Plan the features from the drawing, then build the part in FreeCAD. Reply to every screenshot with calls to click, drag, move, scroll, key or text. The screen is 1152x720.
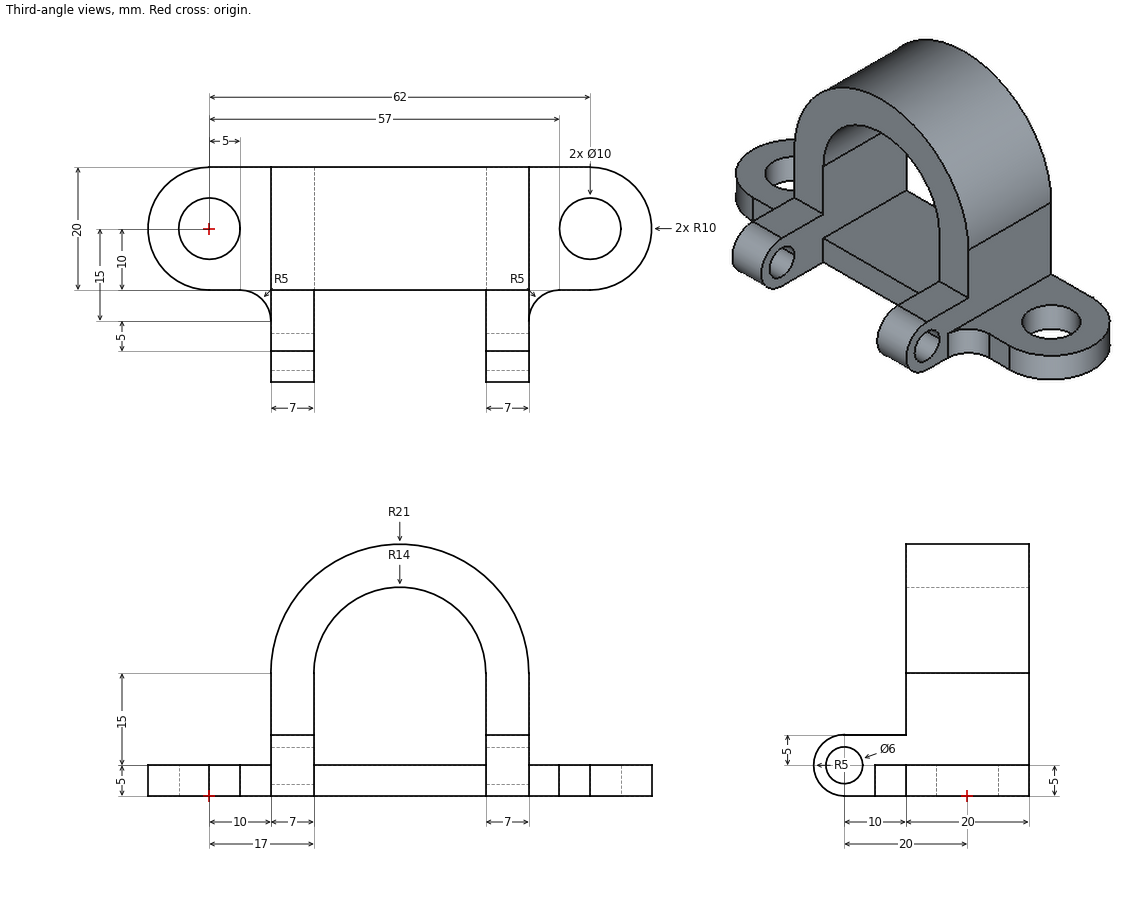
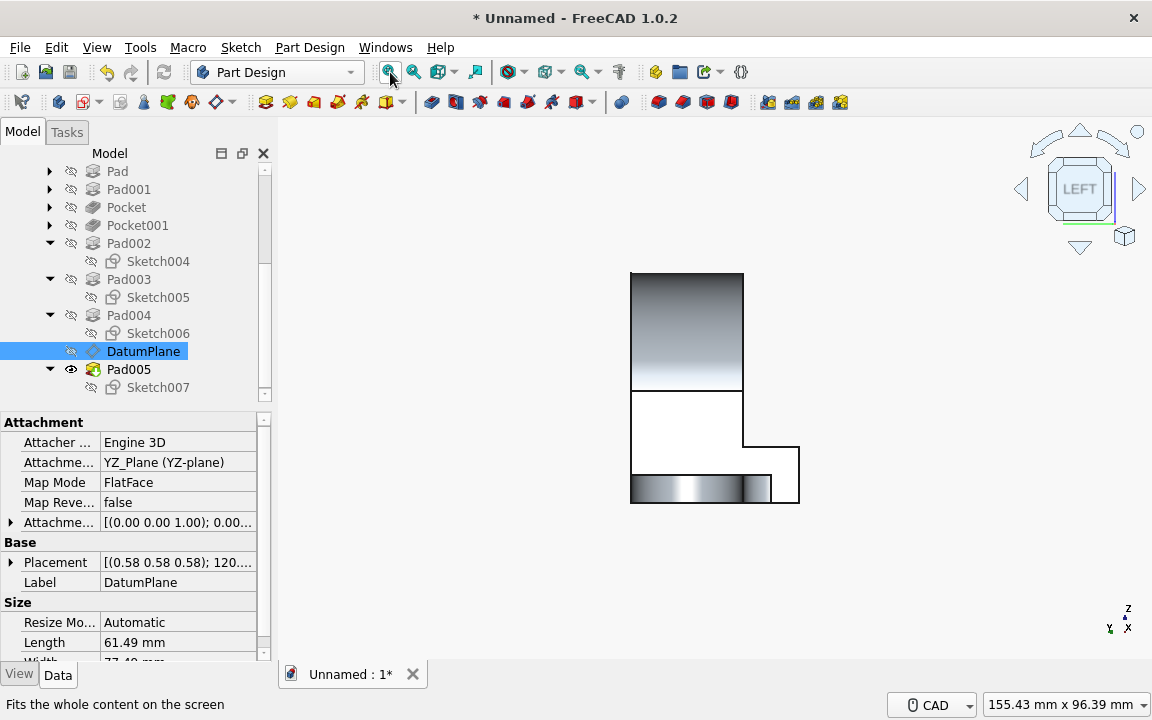
click(691, 430)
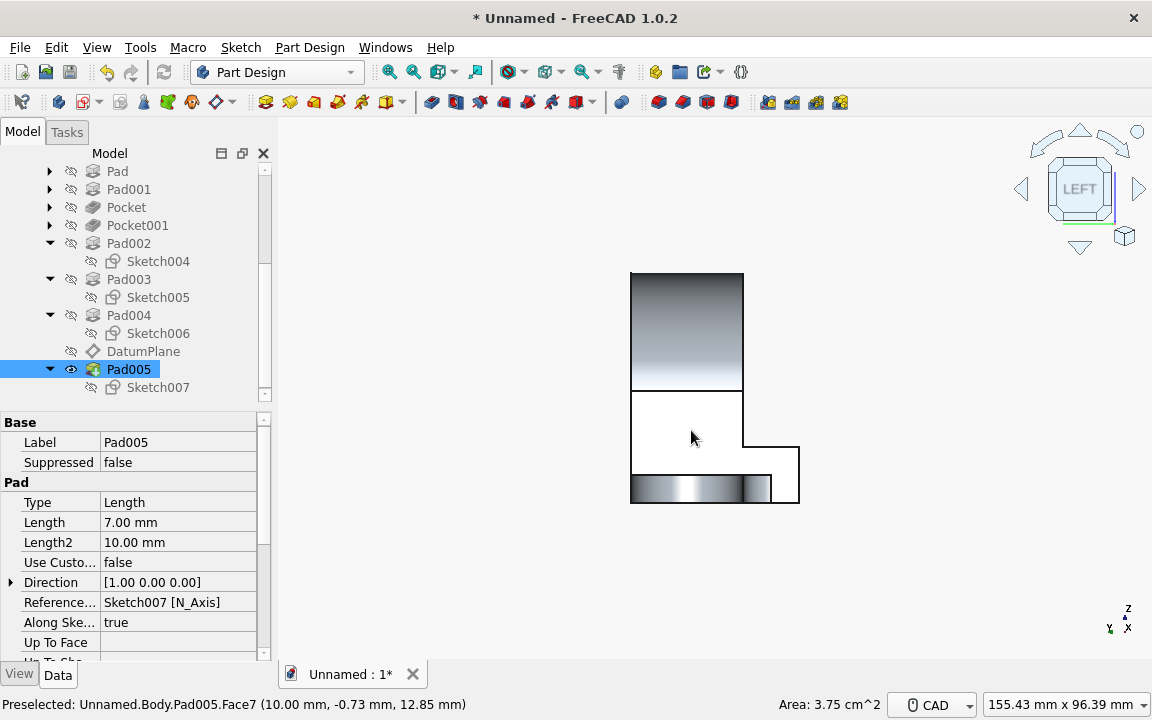
click(84, 102)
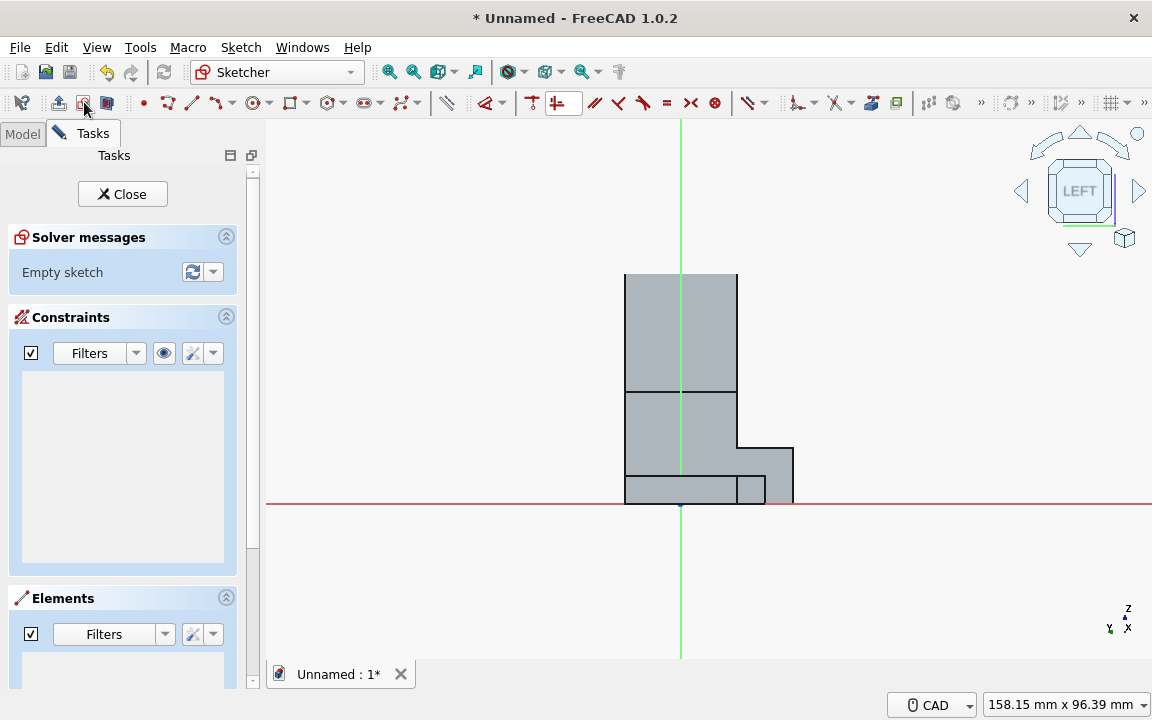
click(108, 104)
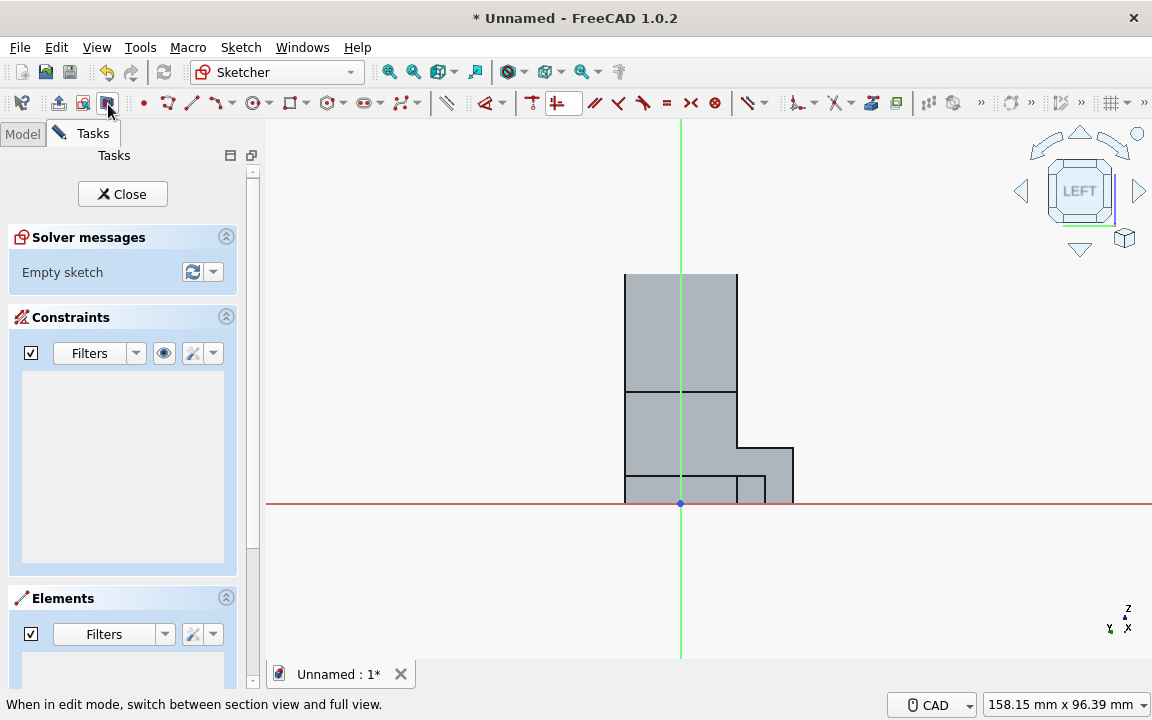
scroll(840, 493, up, 9)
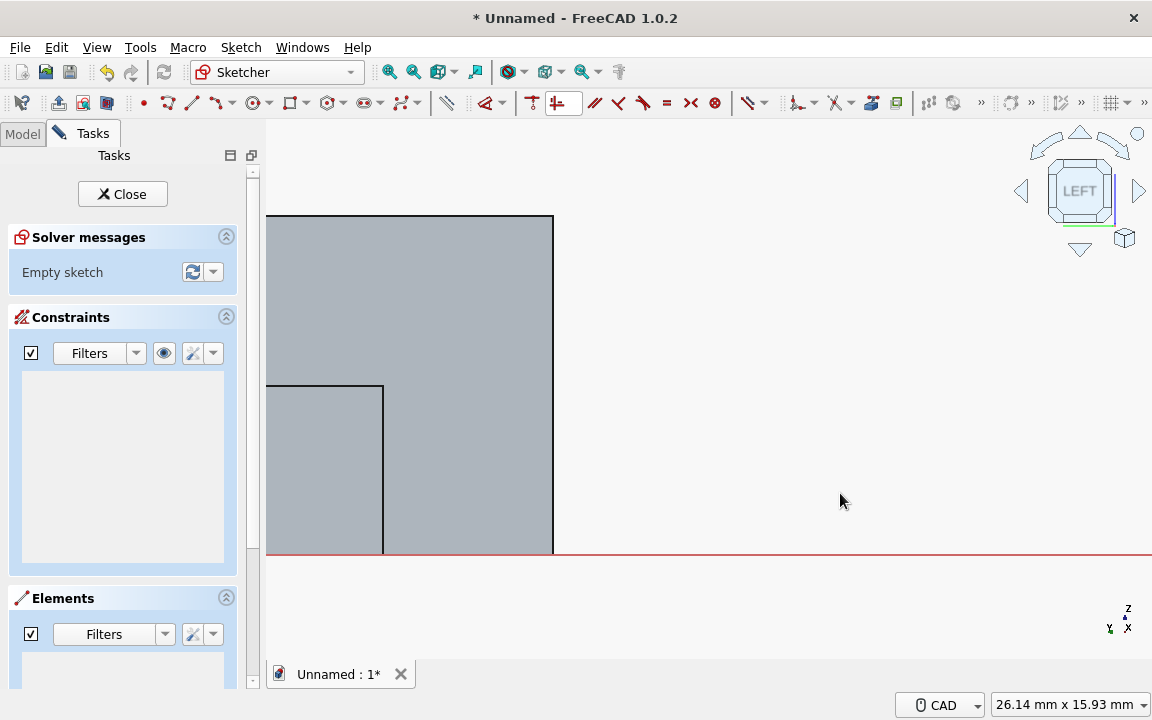
click(192, 104)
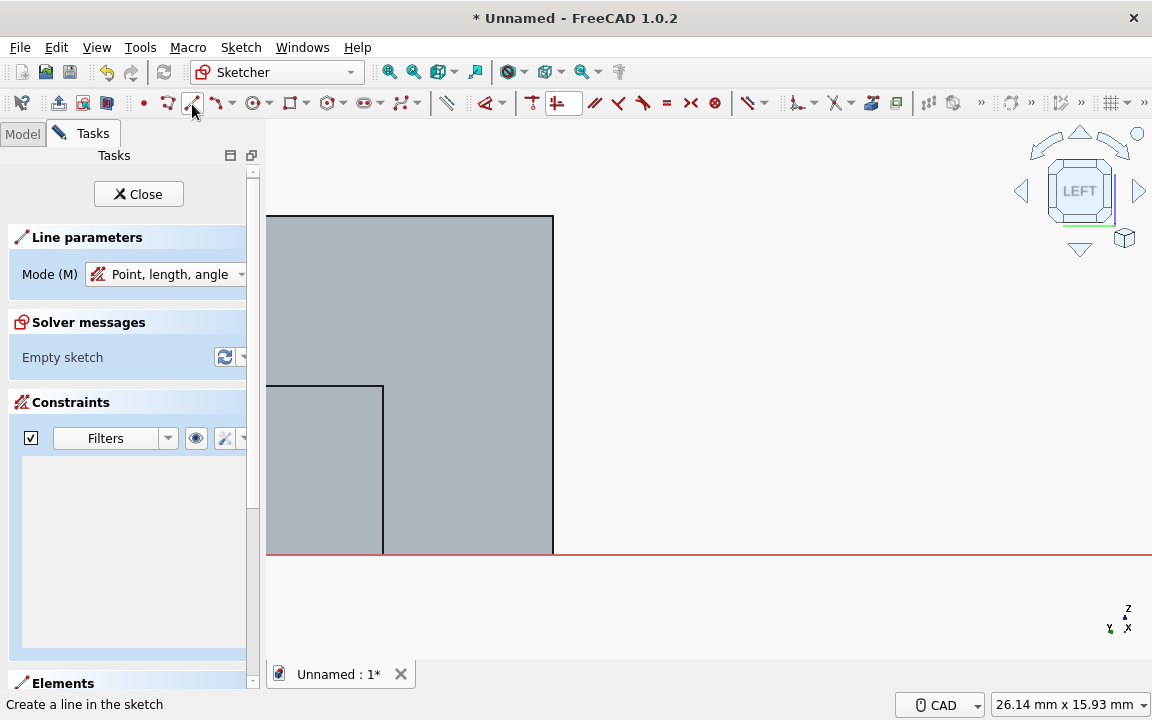
click(553, 216)
click(553, 555)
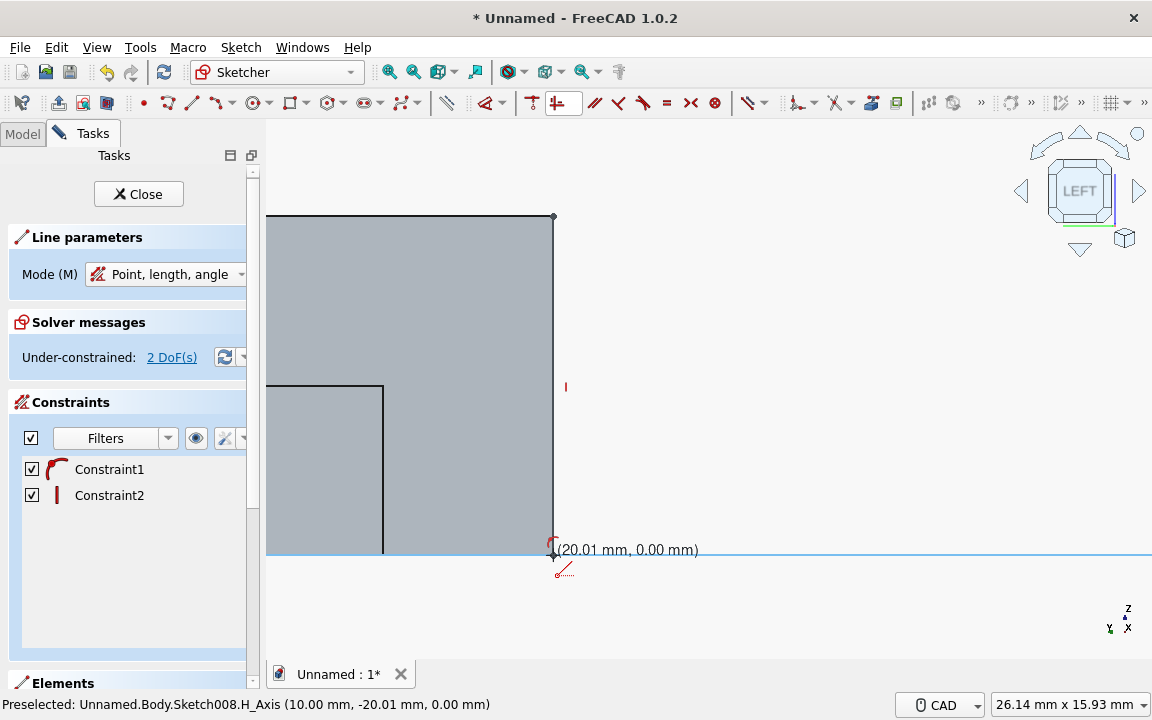
click(216, 104)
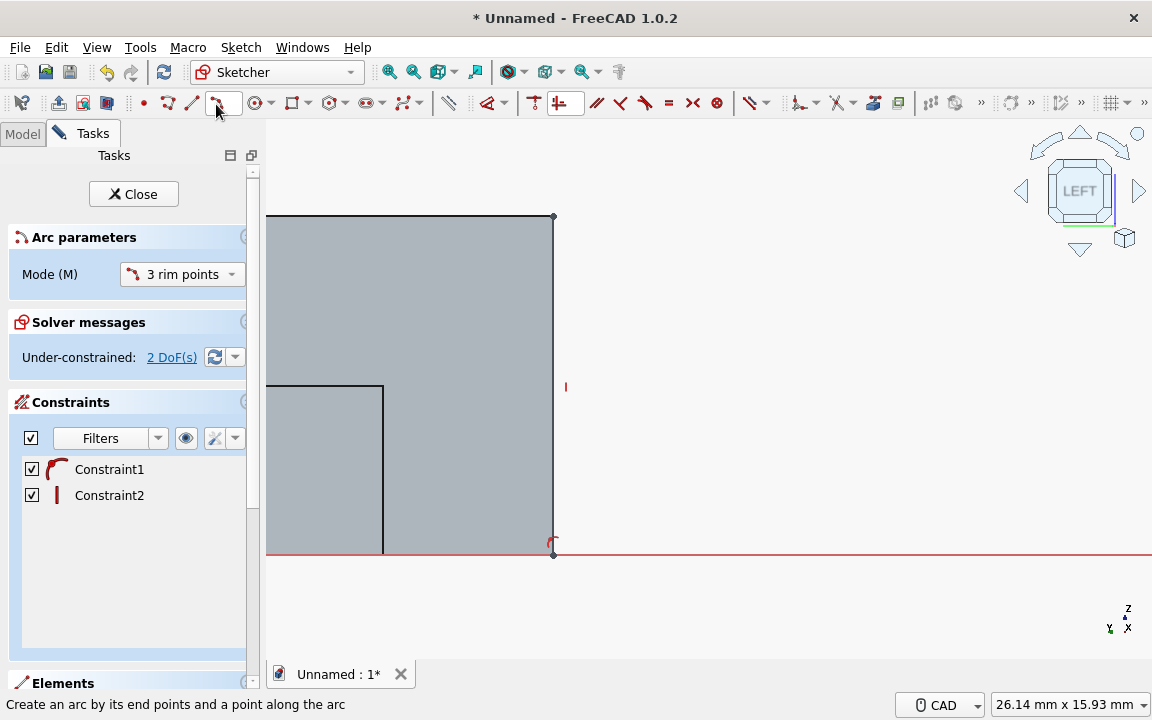
click(553, 555)
click(553, 217)
click(722, 386)
key(Escape)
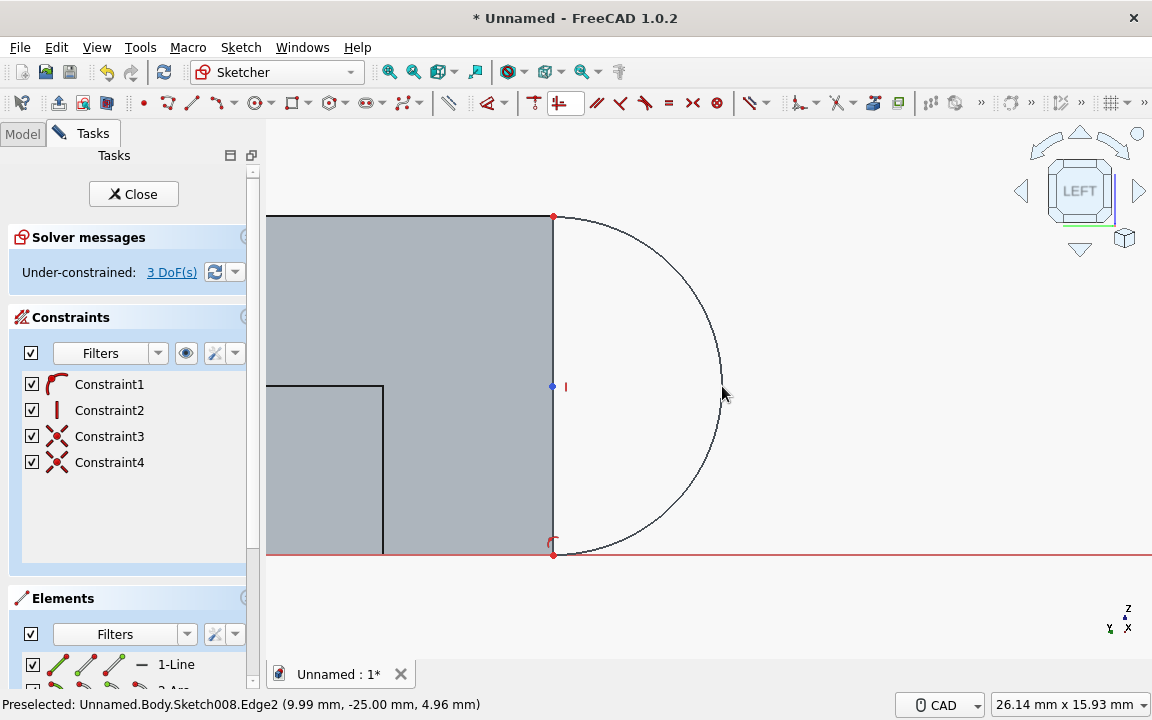
click(488, 104)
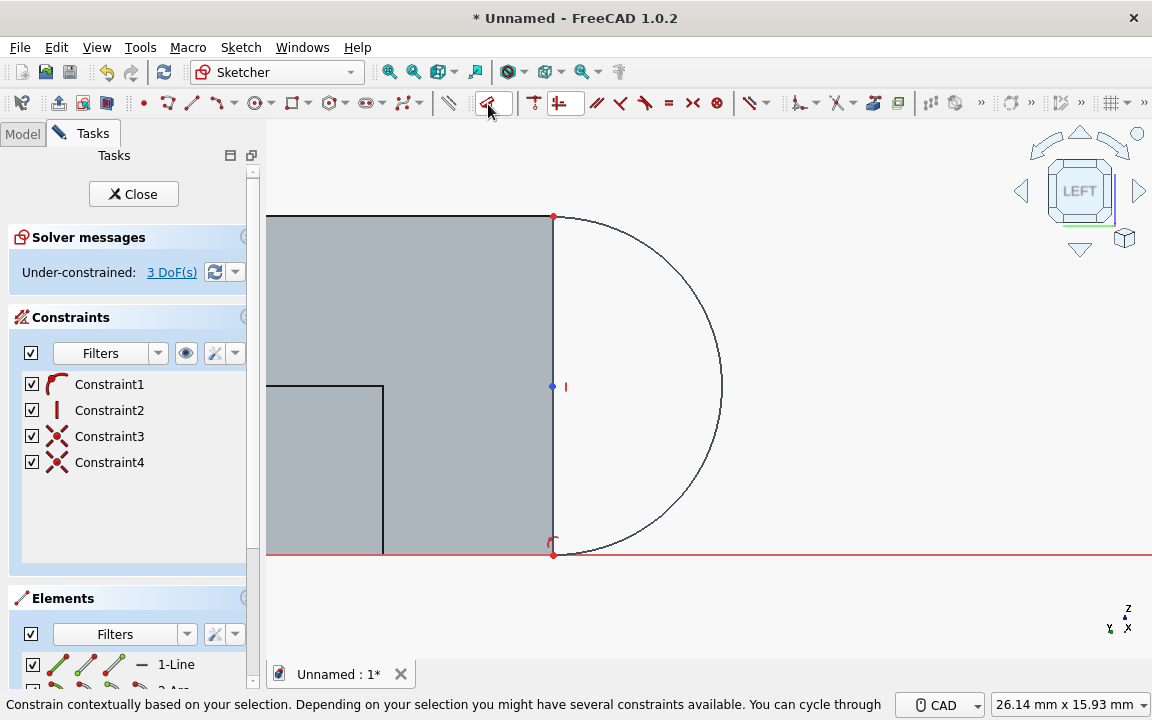
click(690, 485)
click(716, 504)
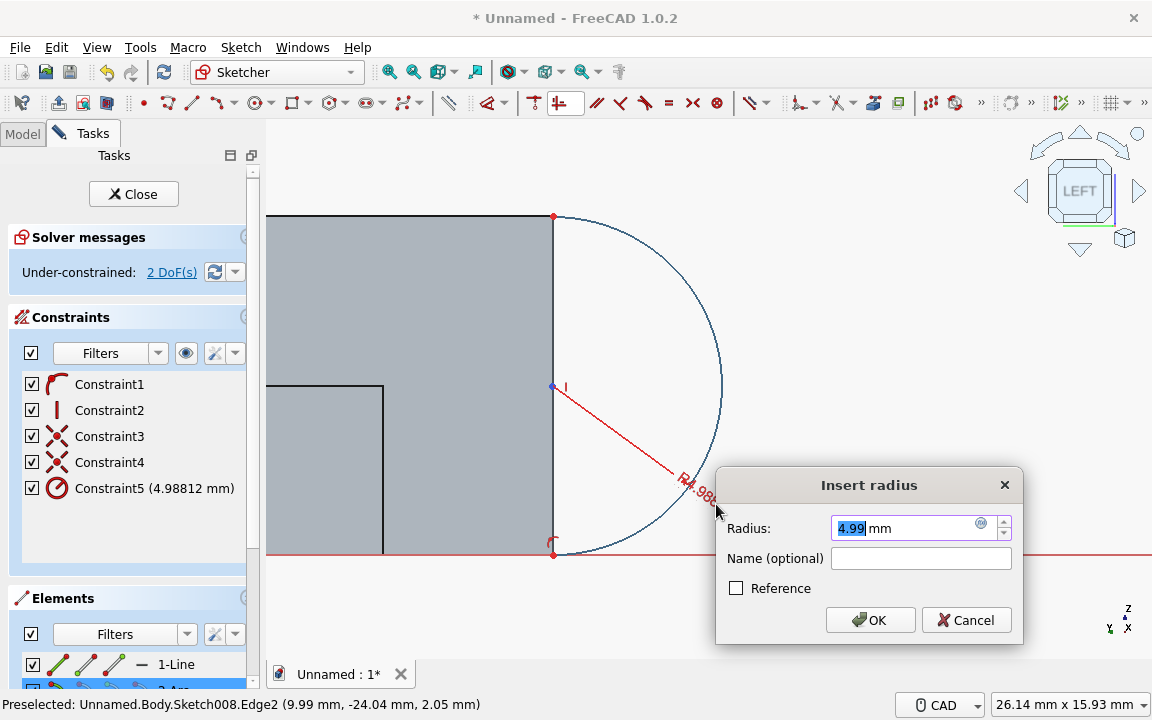
text(5)
key(Return)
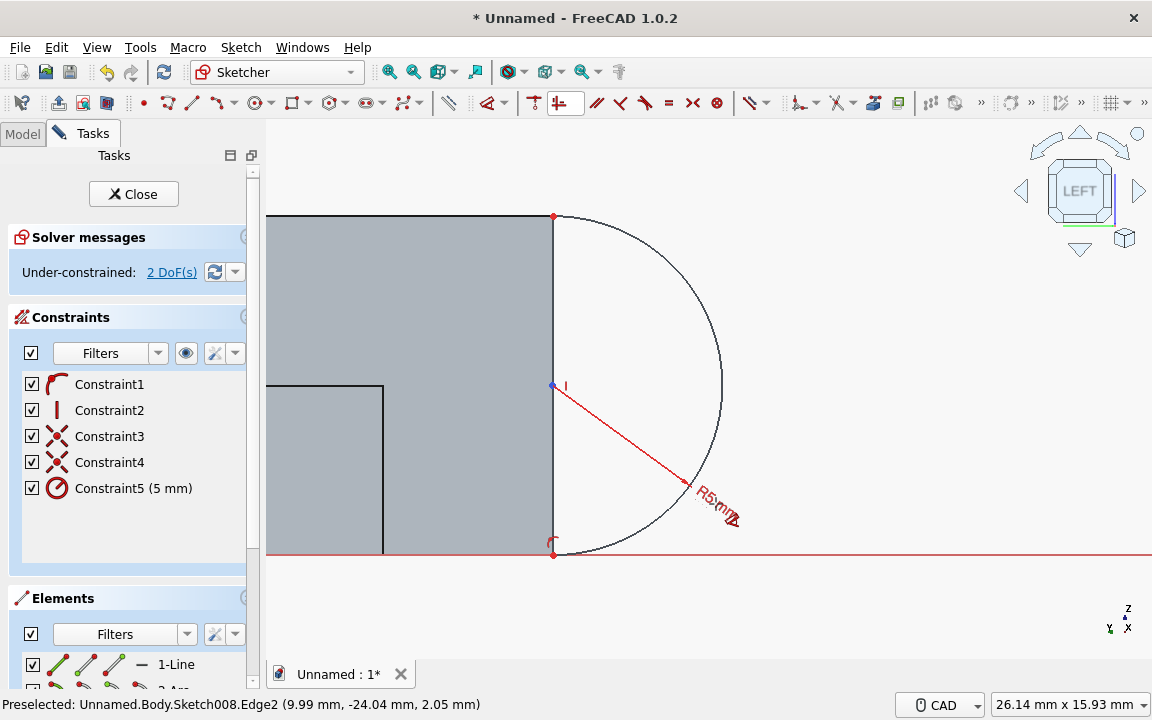
click(553, 216)
click(424, 589)